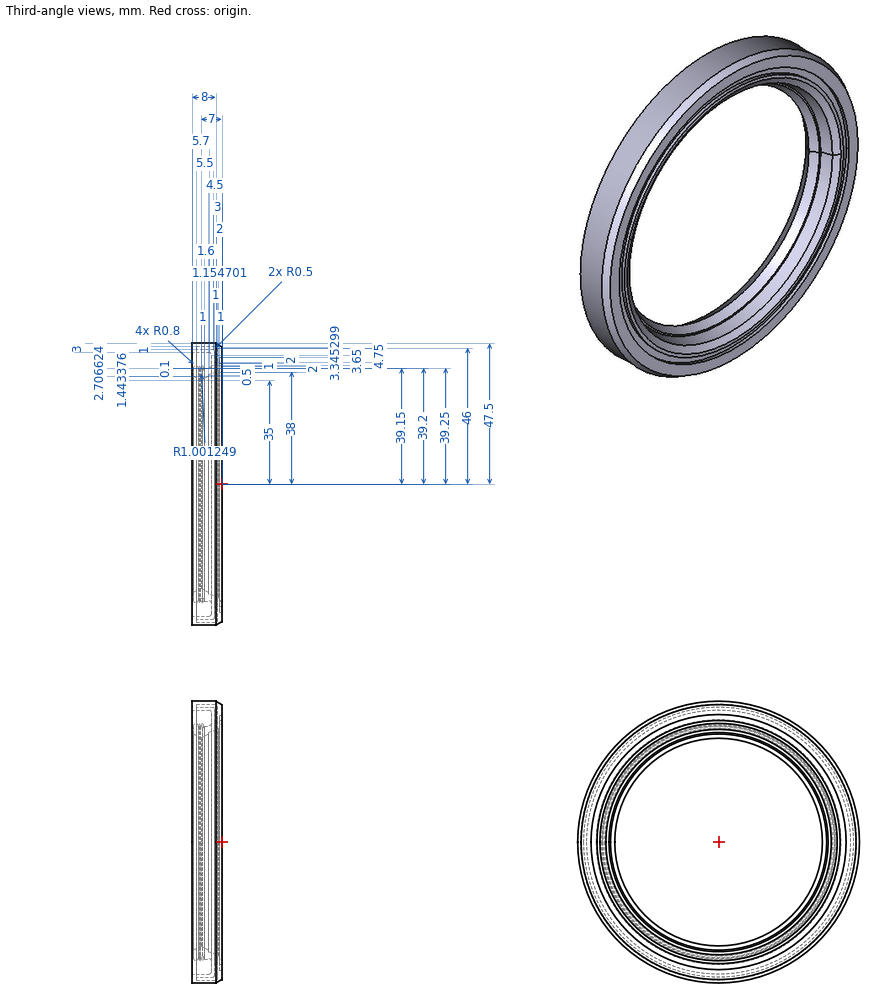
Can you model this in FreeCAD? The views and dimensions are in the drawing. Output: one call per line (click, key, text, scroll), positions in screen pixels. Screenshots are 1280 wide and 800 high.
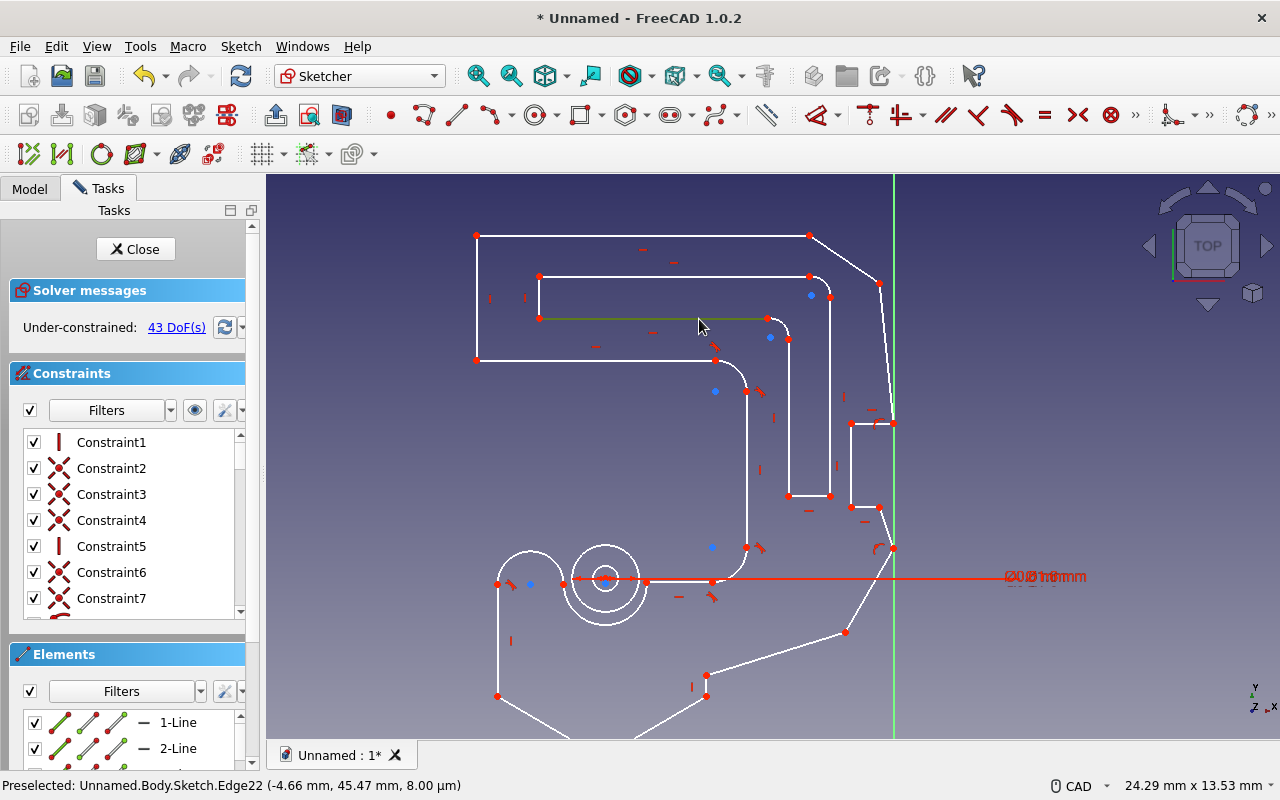
scroll(787, 329, up, 2)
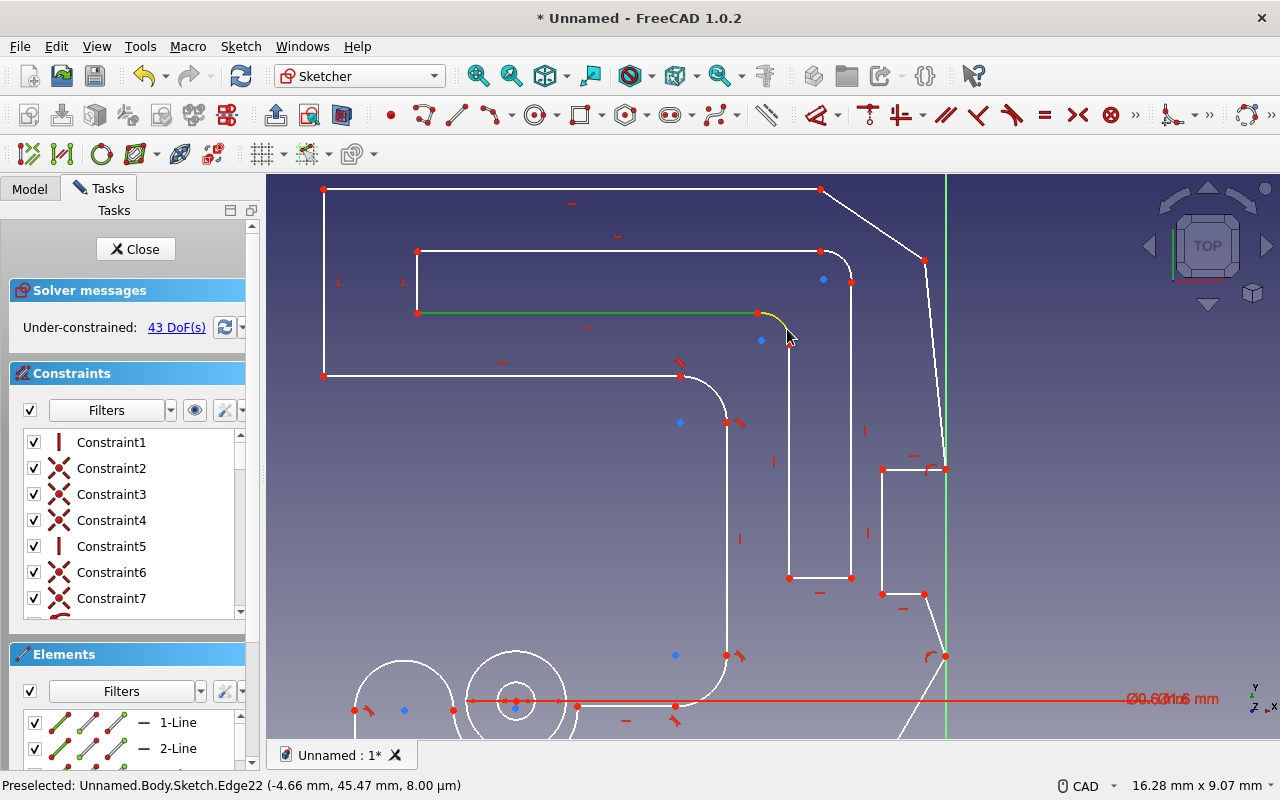
click(787, 330)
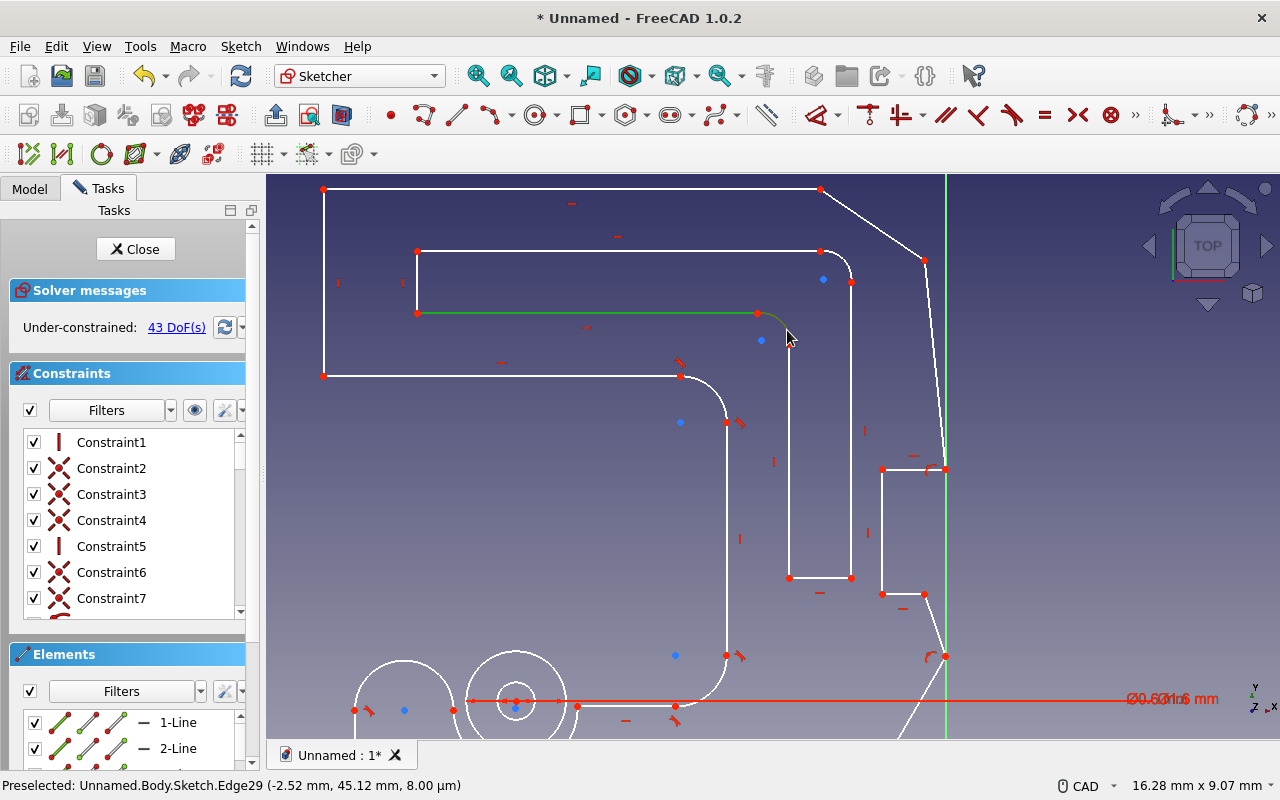
click(1012, 116)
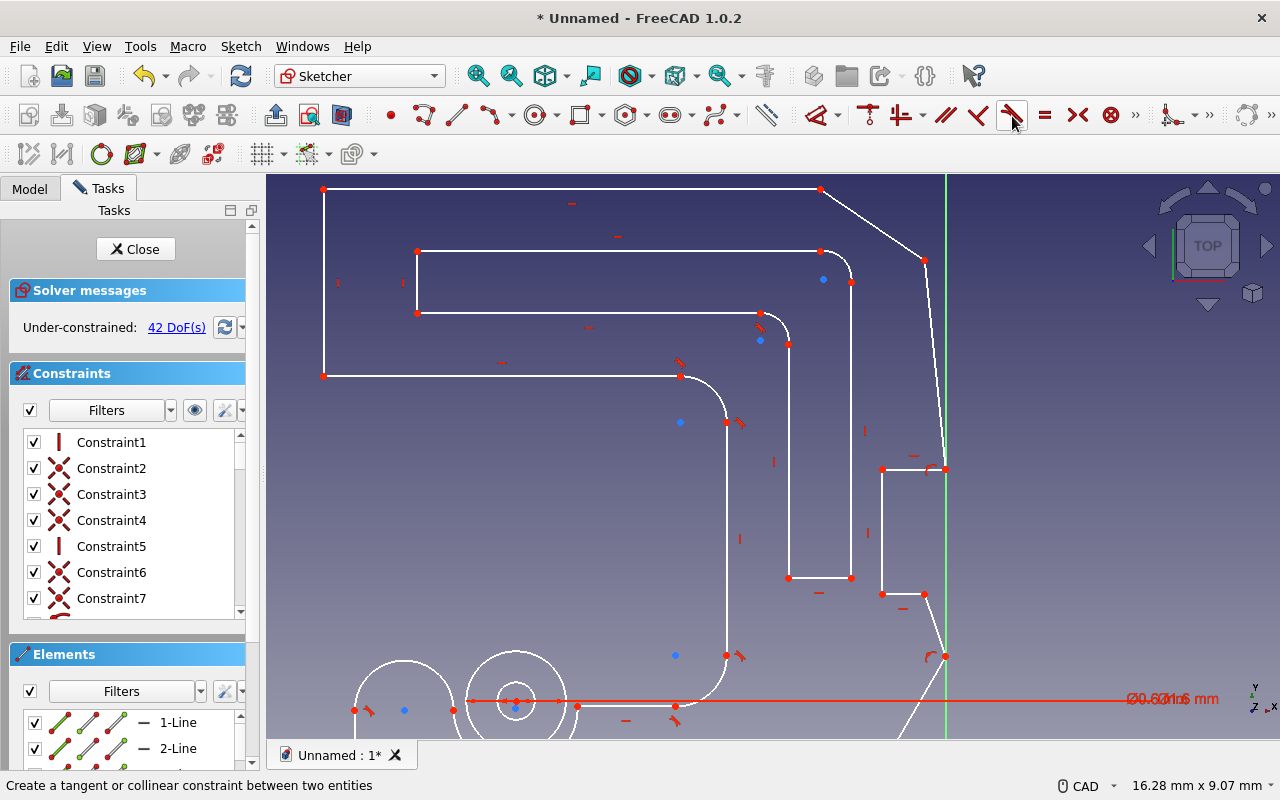
click(538, 251)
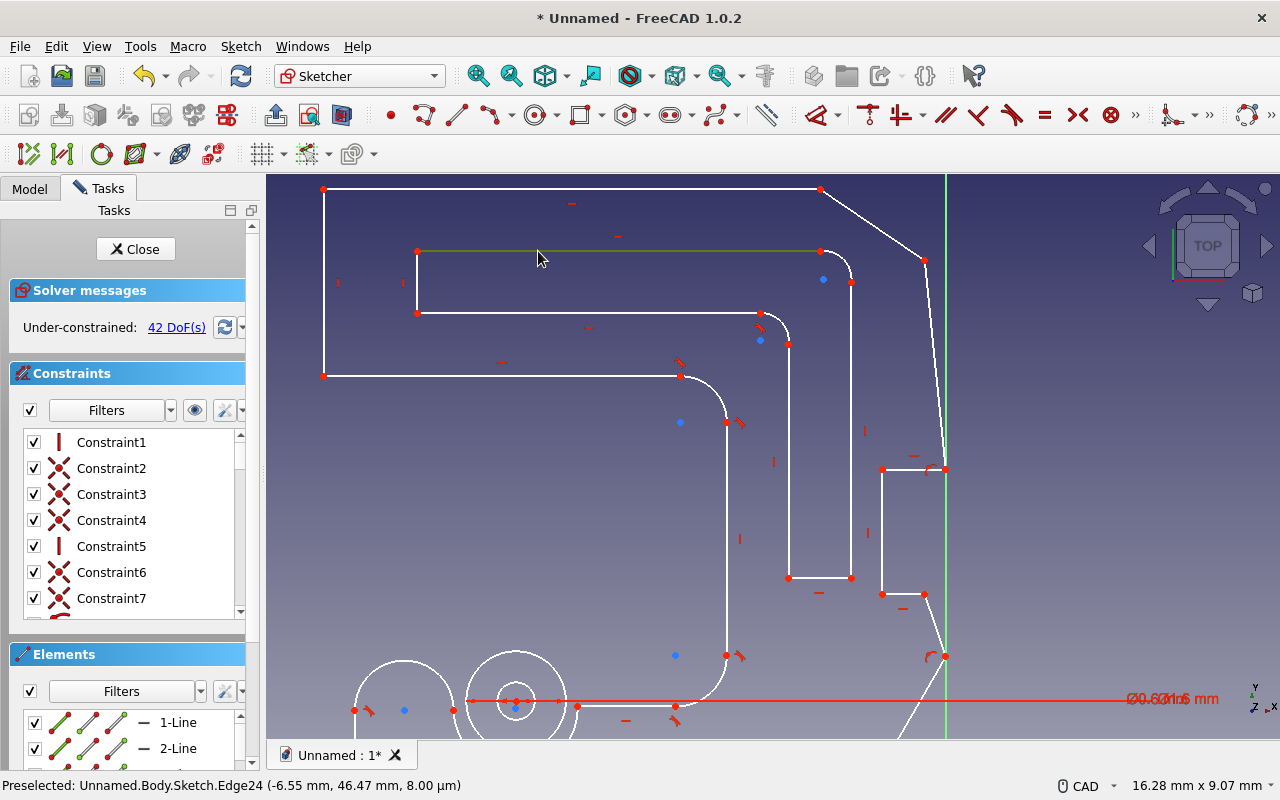
click(849, 267)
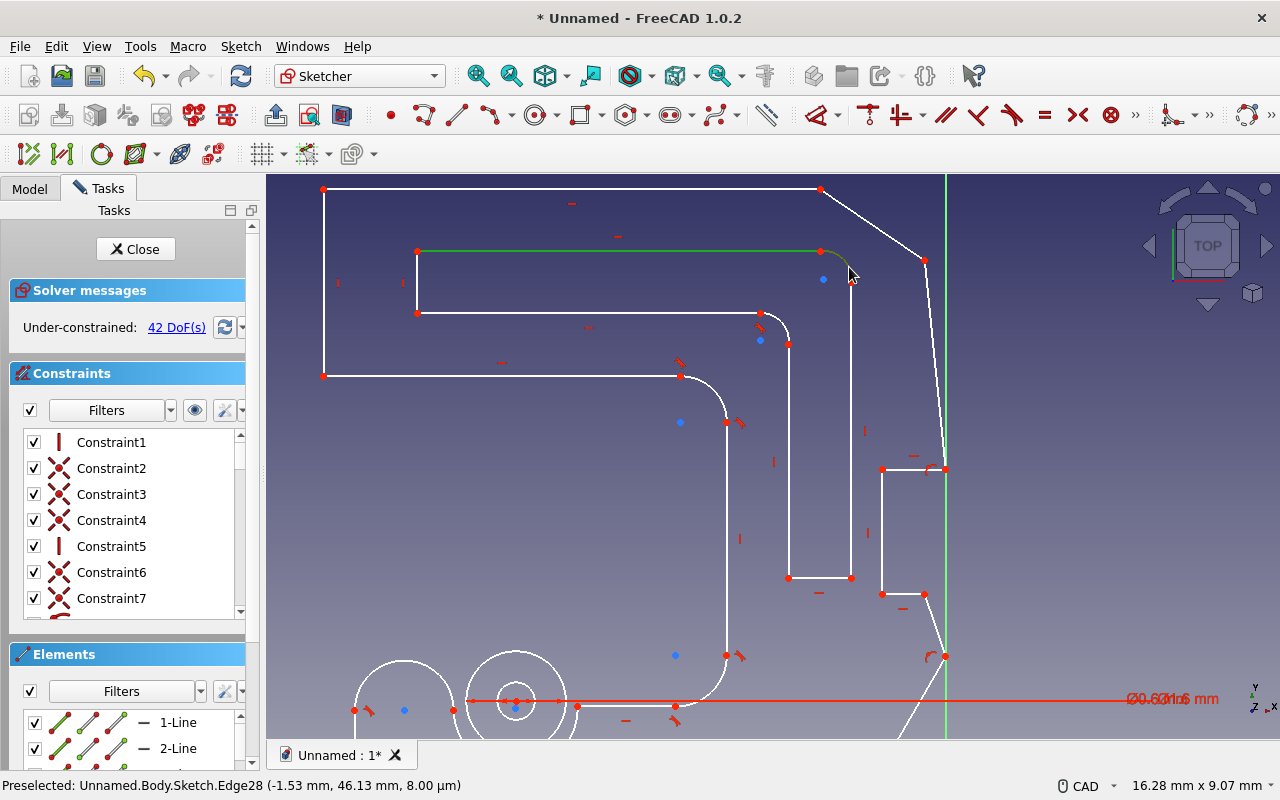
click(1012, 116)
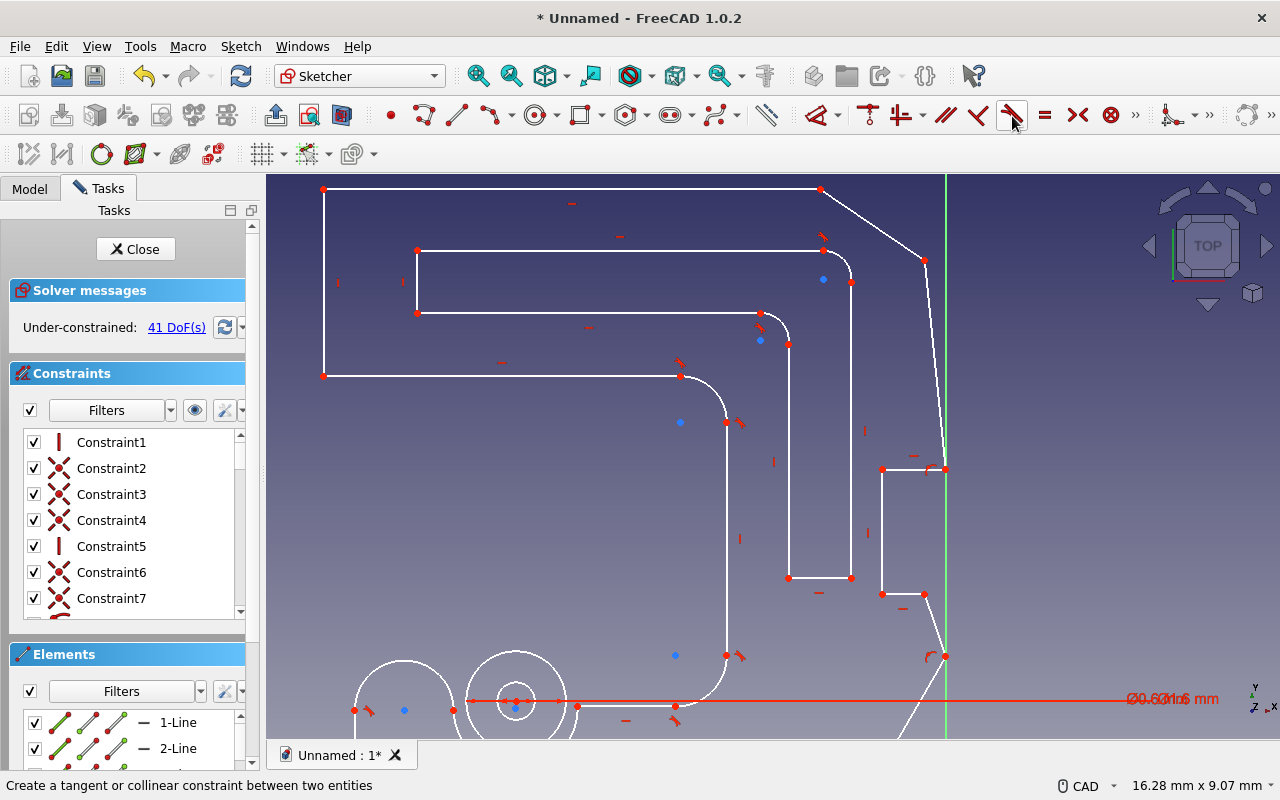
click(851, 371)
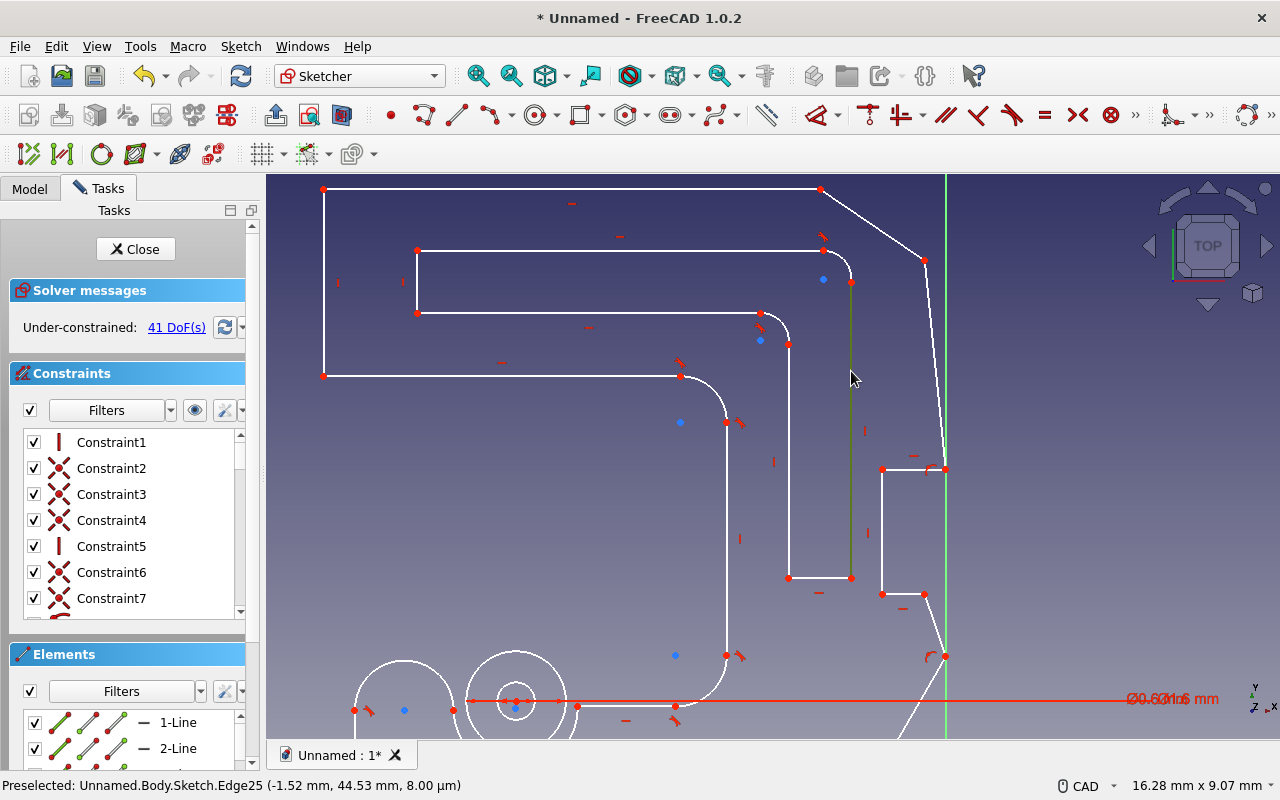
click(849, 268)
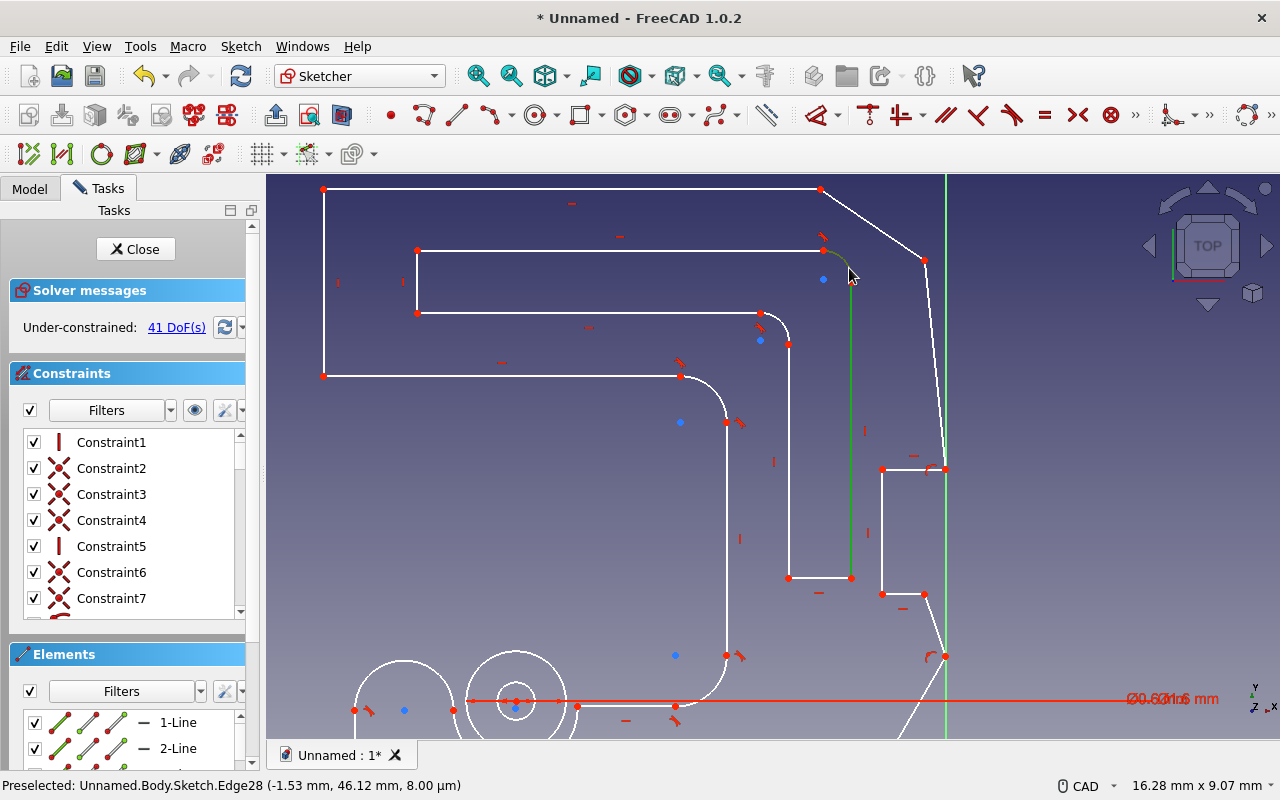
key(t)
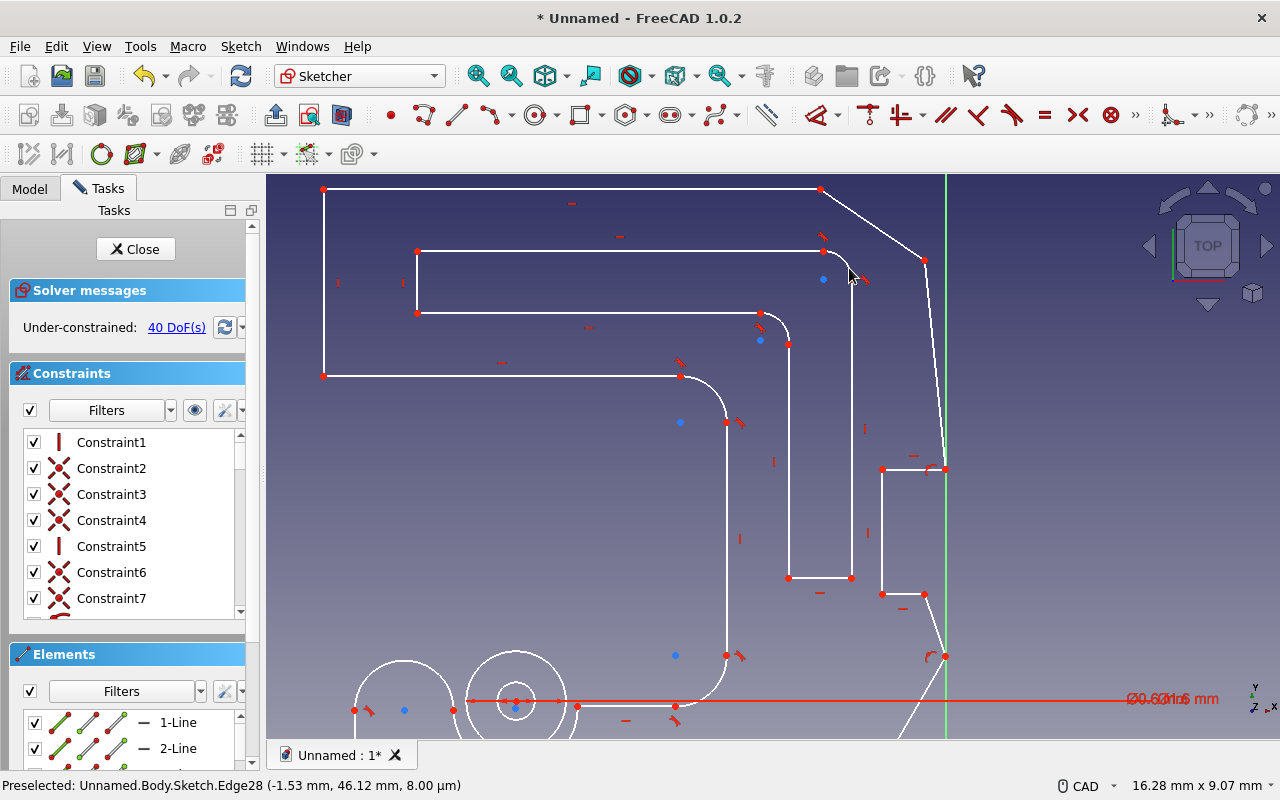
click(789, 508)